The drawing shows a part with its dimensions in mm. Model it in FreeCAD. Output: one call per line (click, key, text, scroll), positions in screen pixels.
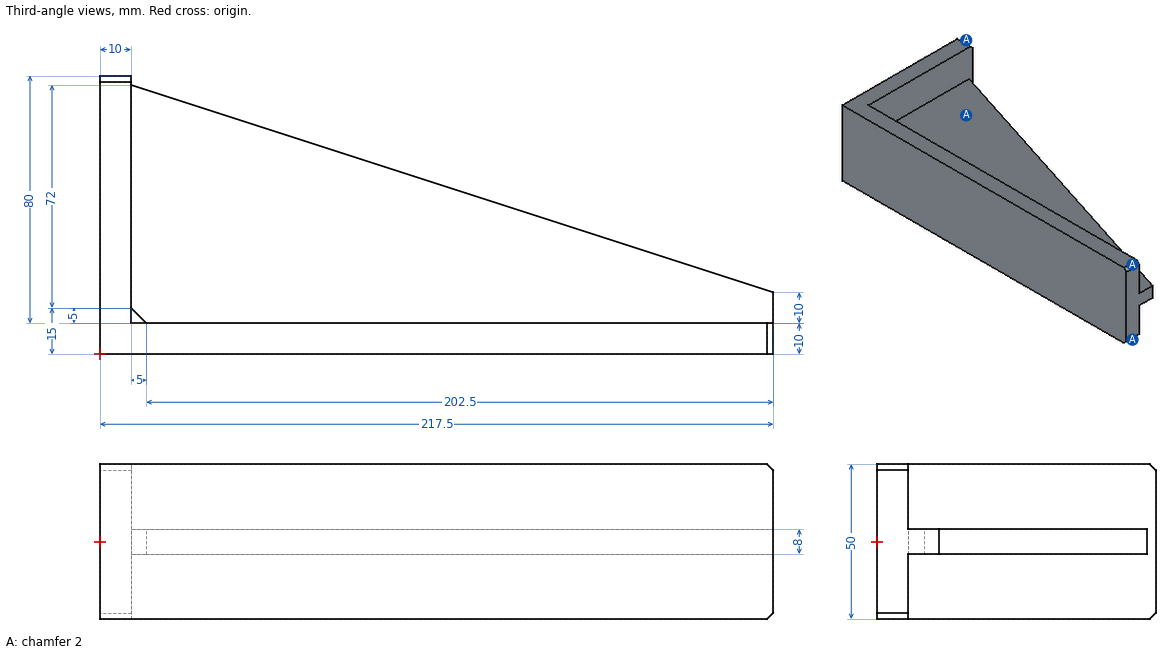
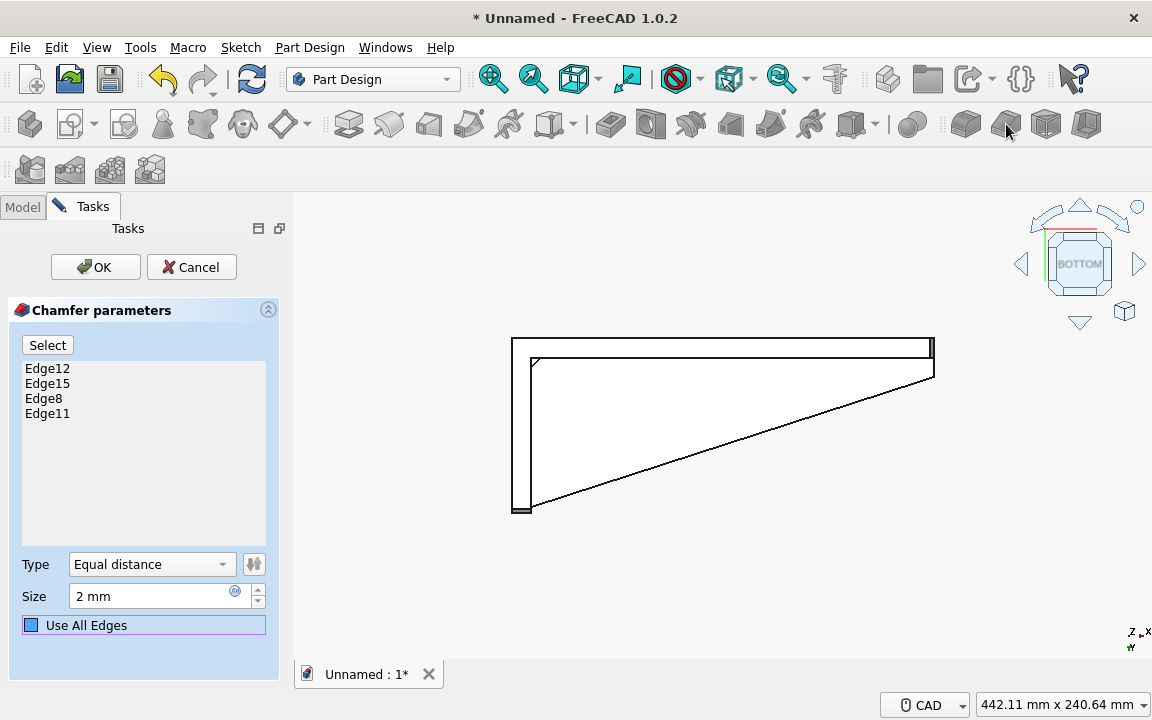
click(96, 267)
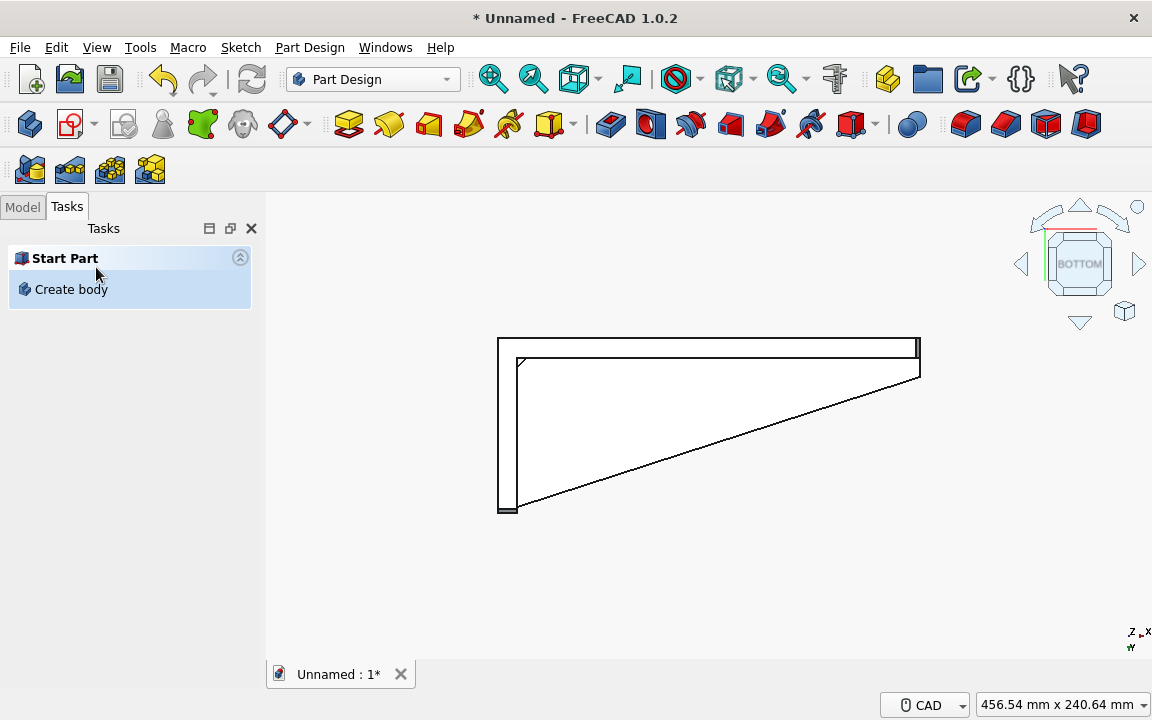
key(0)